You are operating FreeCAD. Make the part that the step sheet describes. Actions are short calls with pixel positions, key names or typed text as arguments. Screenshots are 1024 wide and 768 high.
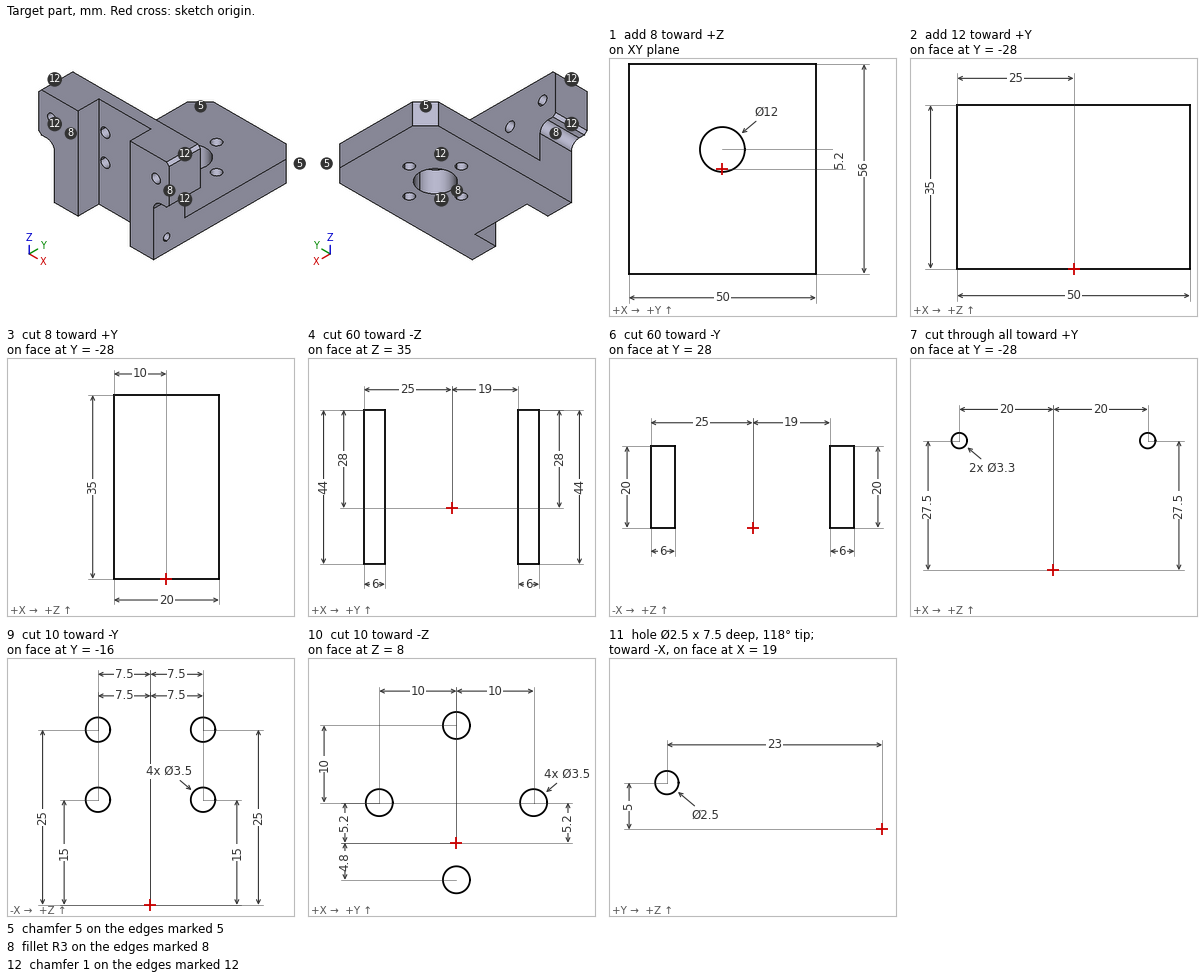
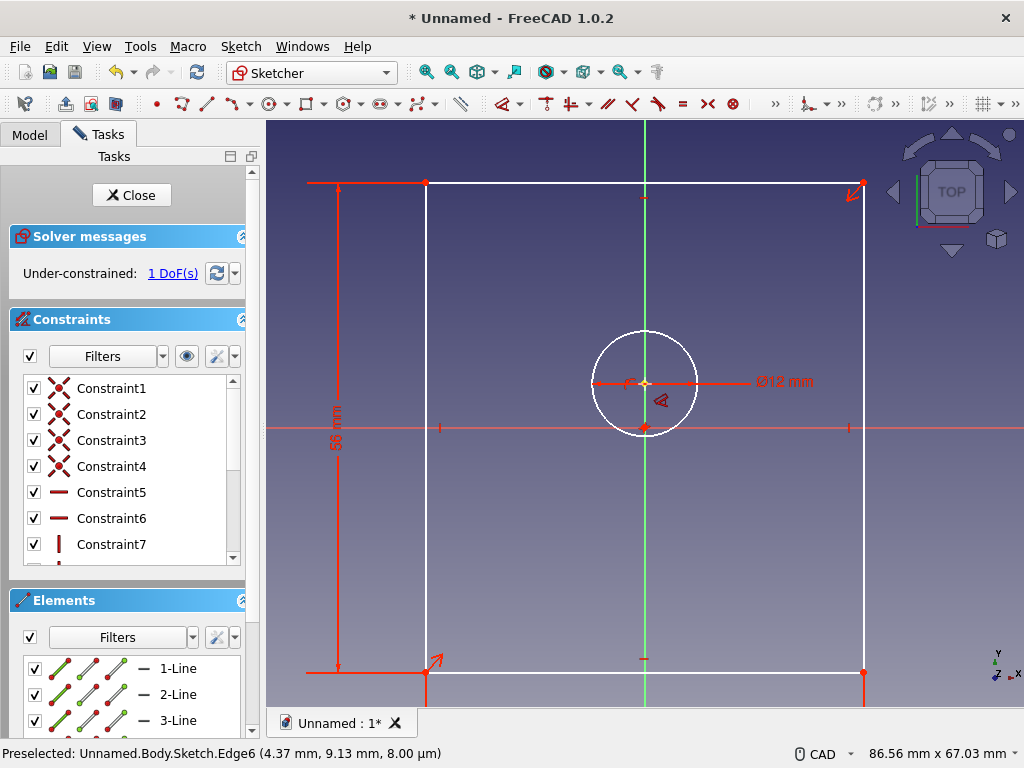
click(645, 384)
click(679, 396)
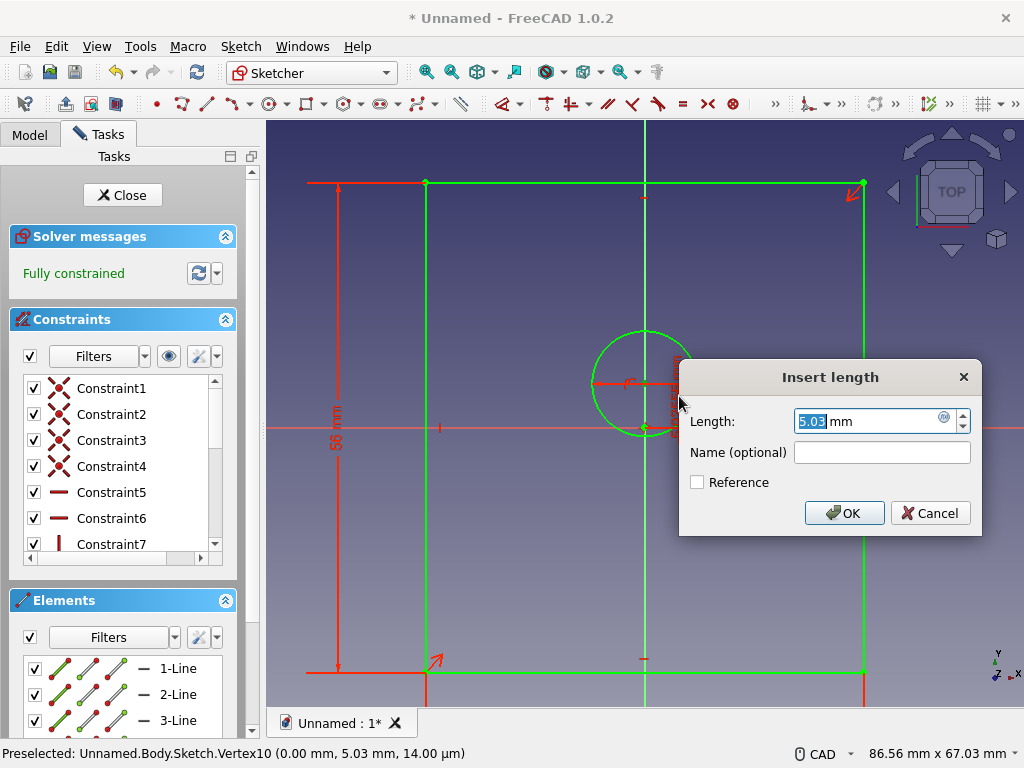
text(5.2)
key(Return)
key(Escape)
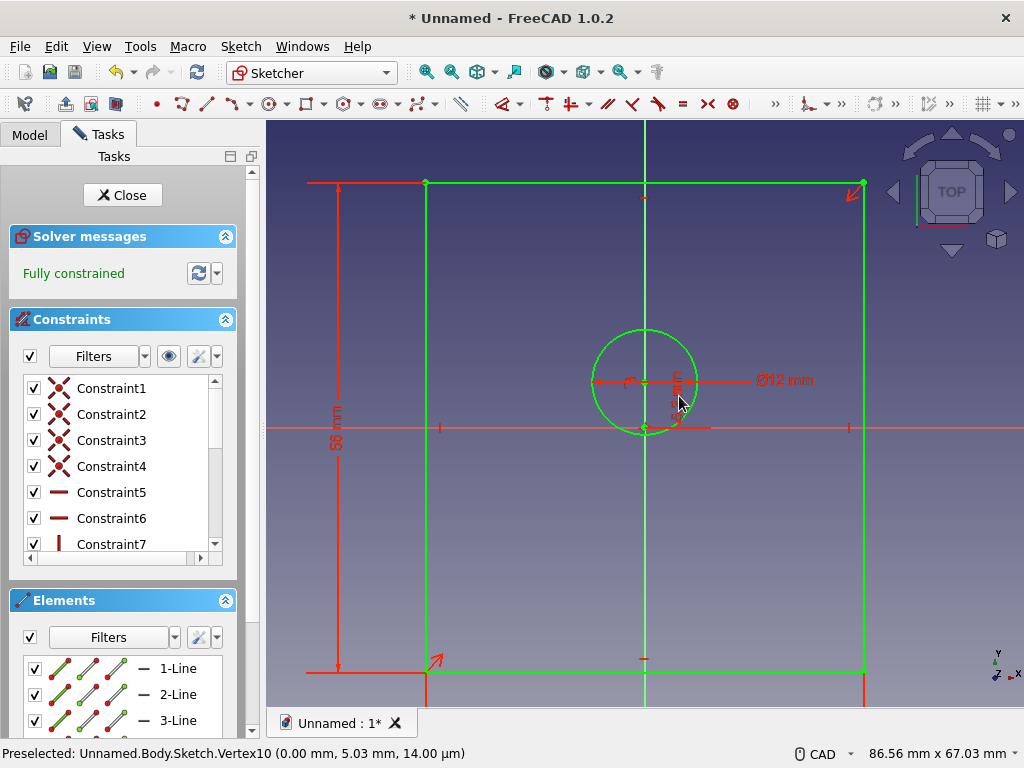
click(123, 195)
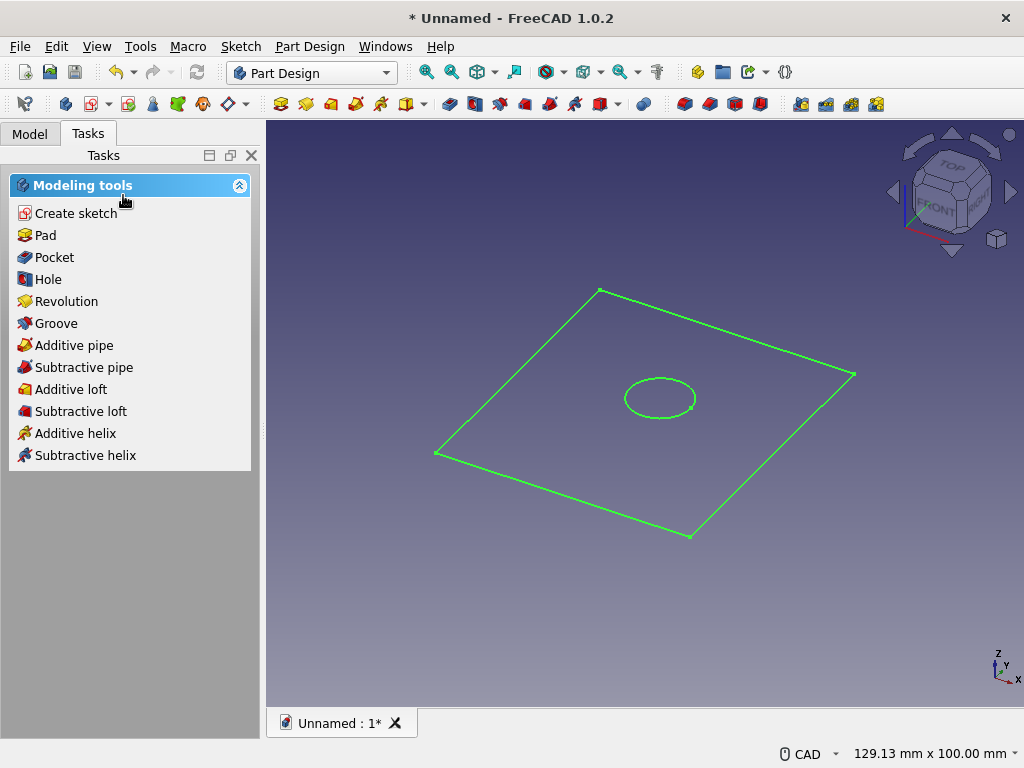
click(281, 104)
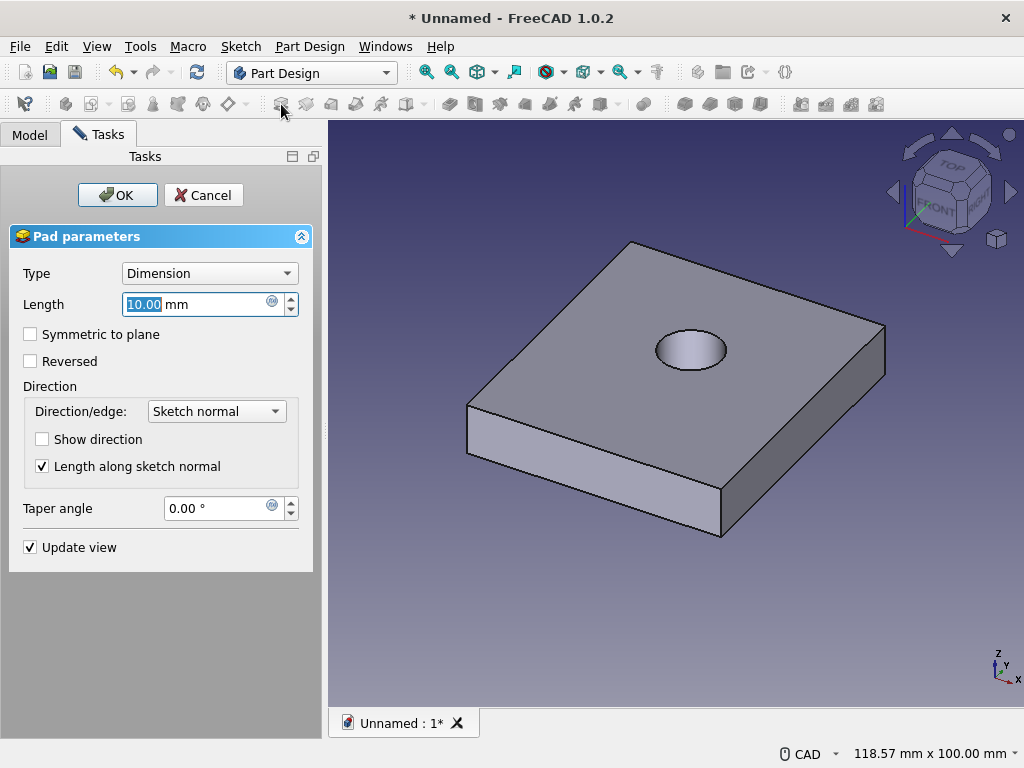
text(8)
key(Tab)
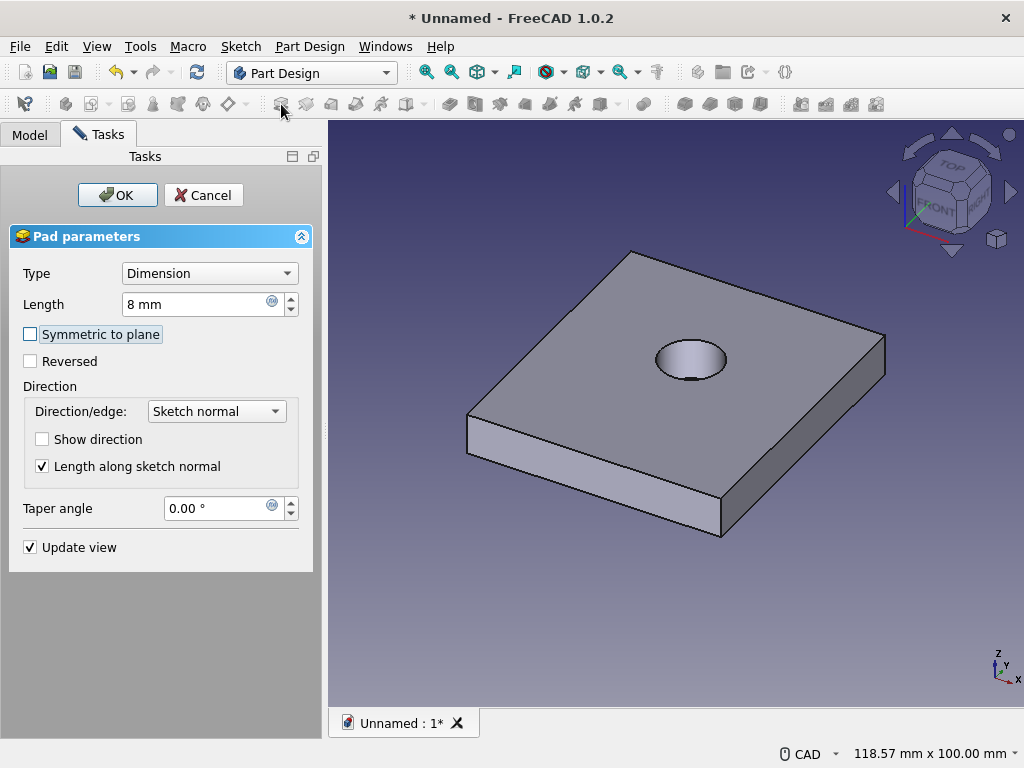
click(118, 195)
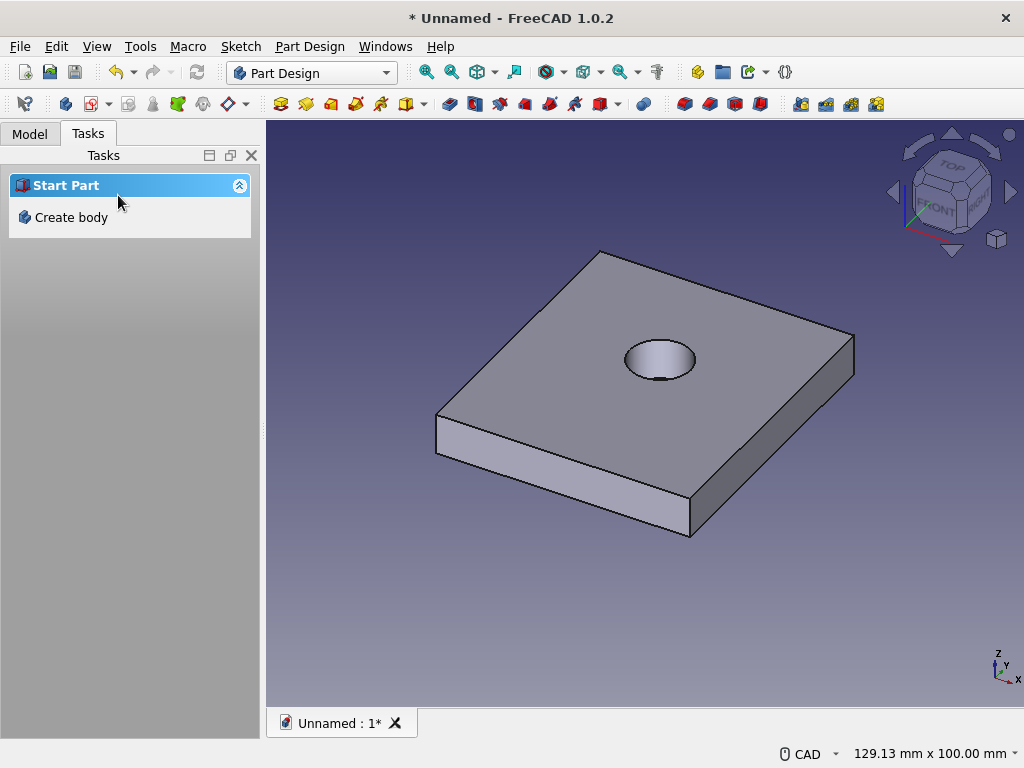
click(635, 499)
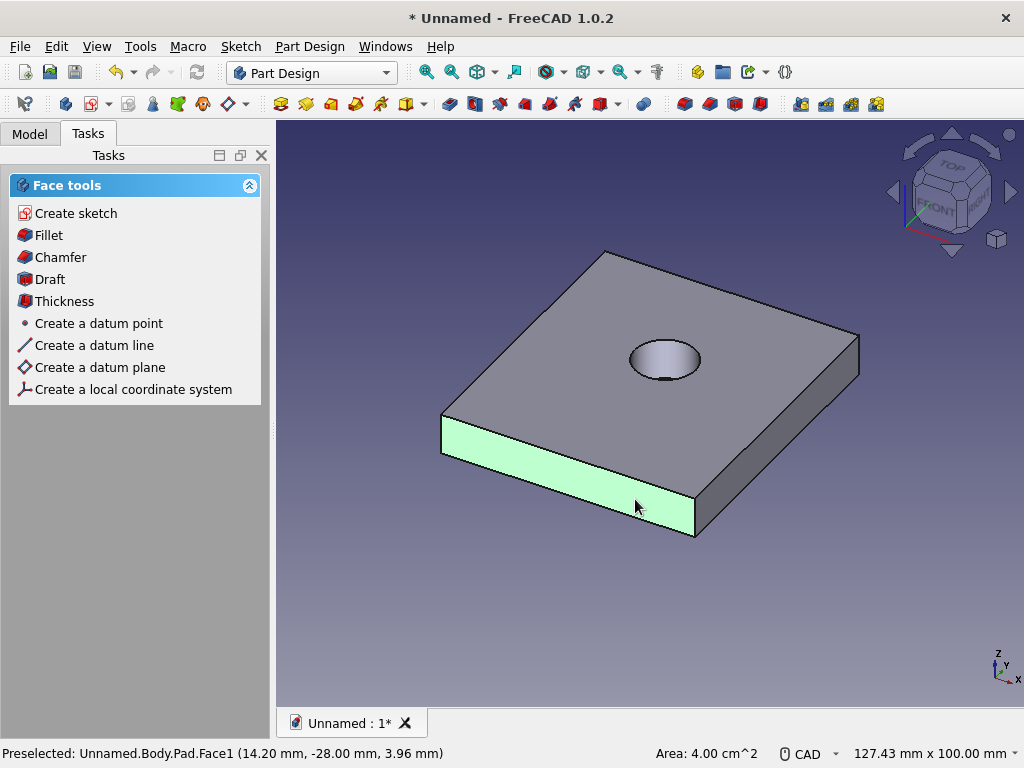
click(90, 104)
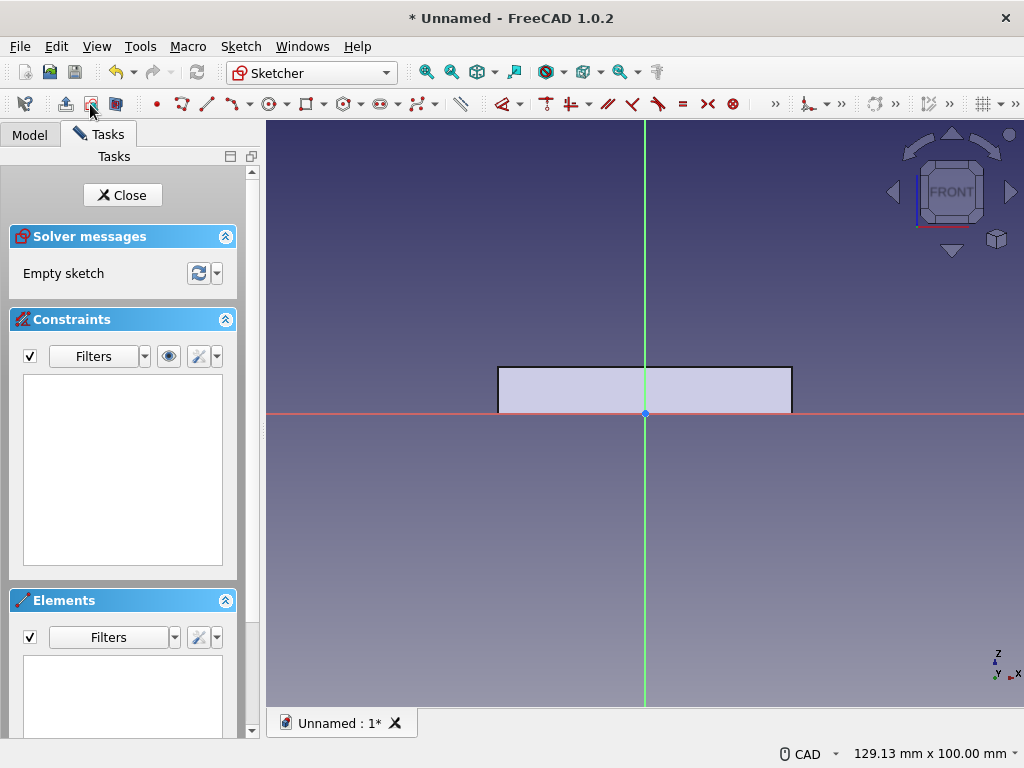
scroll(784, 148, up, 2)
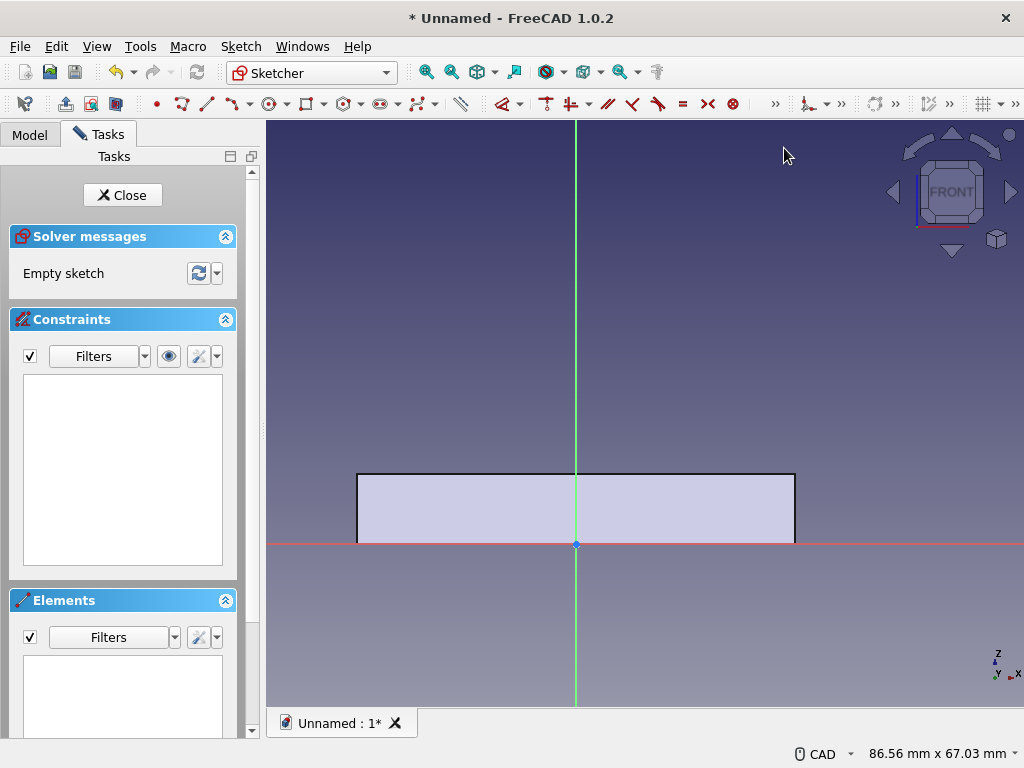
click(306, 104)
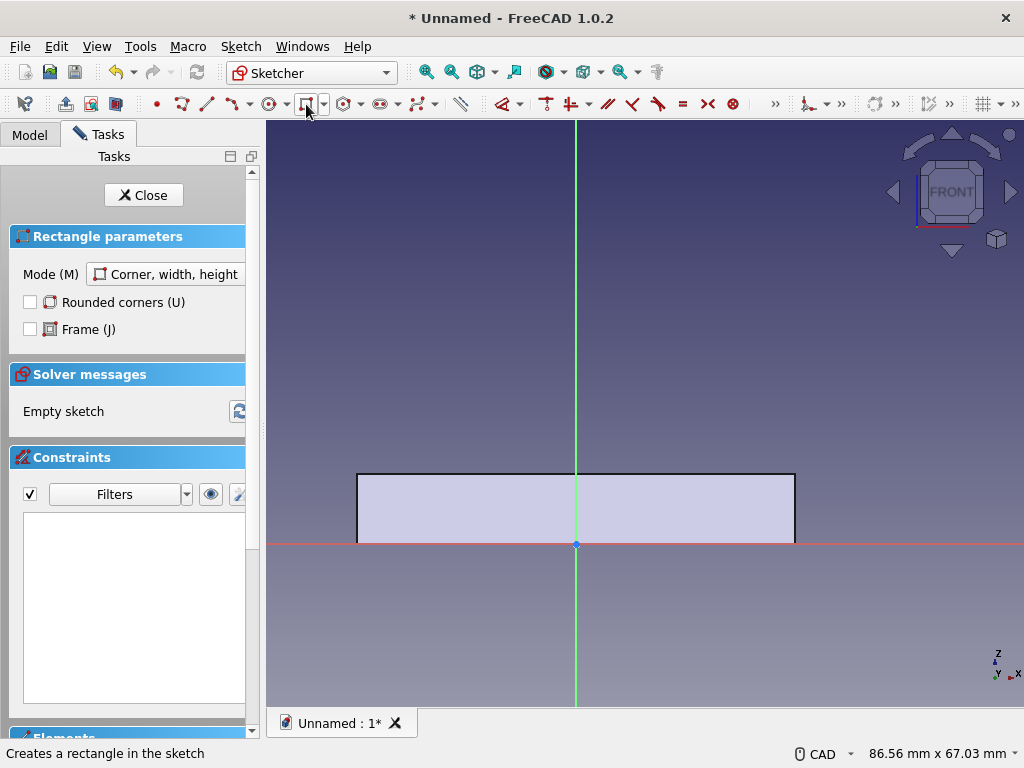
click(357, 238)
click(795, 544)
key(Escape)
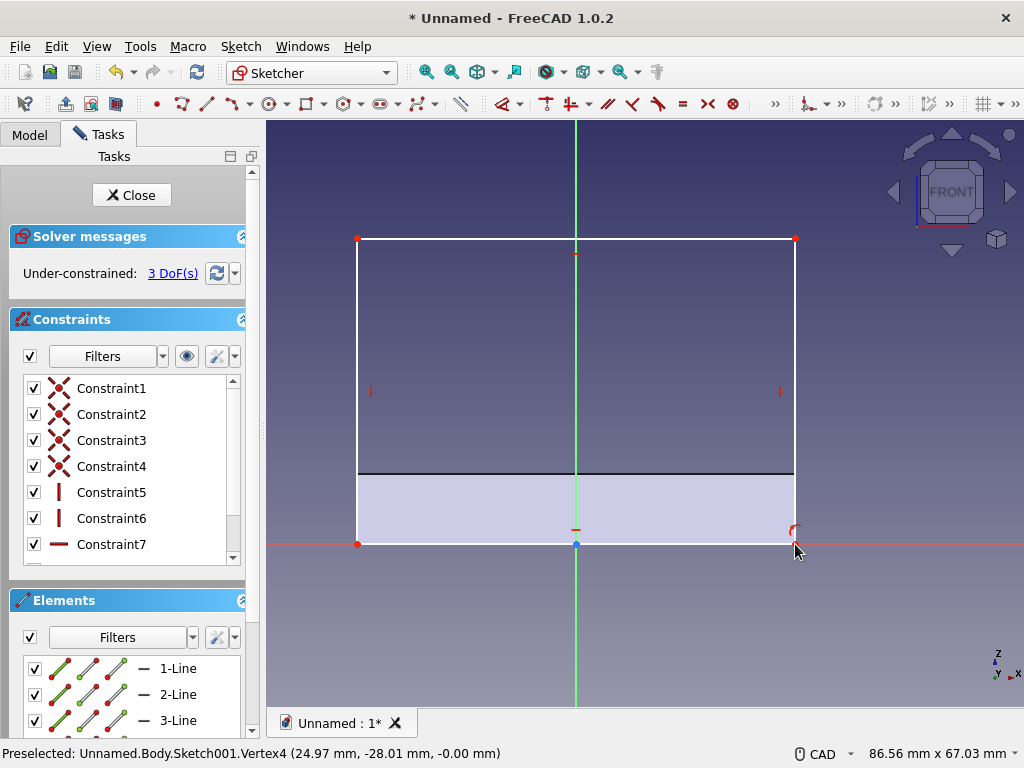
click(502, 104)